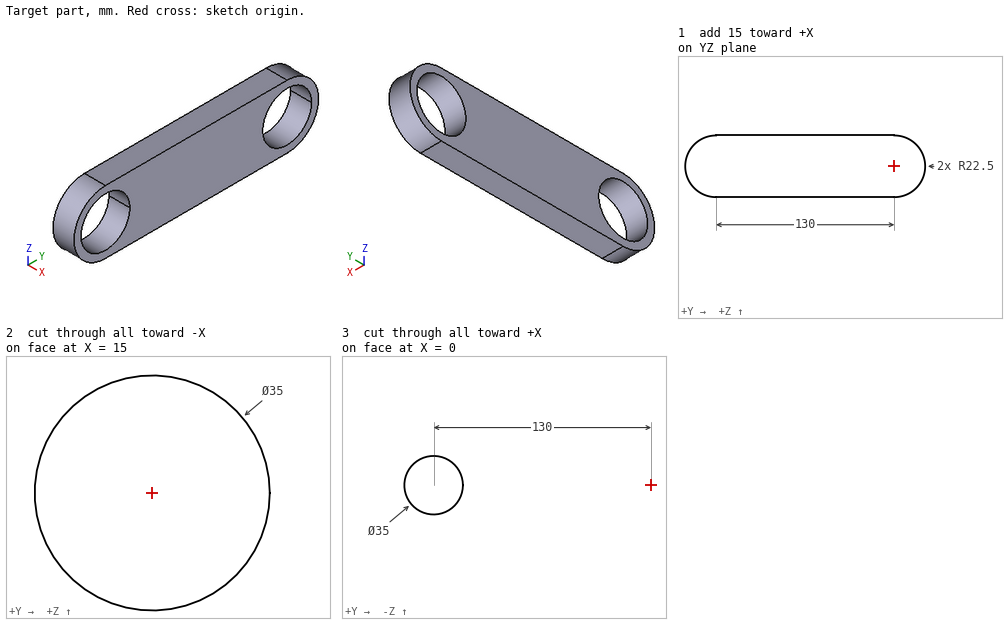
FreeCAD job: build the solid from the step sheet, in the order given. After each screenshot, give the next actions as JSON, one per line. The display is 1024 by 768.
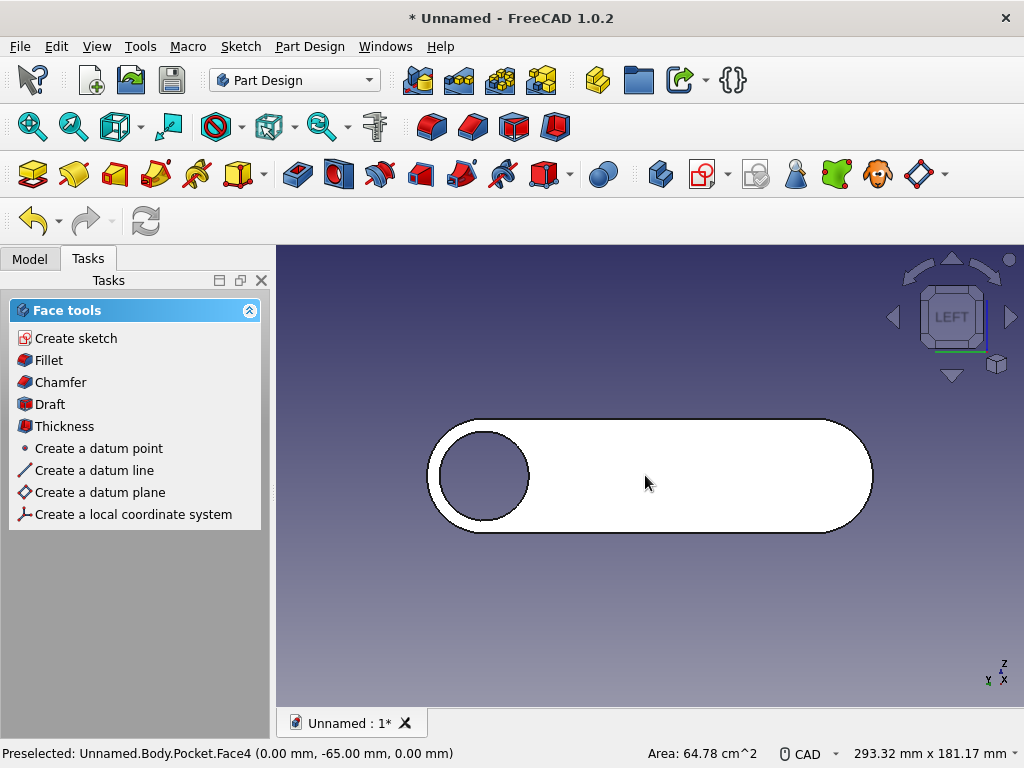
{"action": "left_click", "coordinate": [702, 174]}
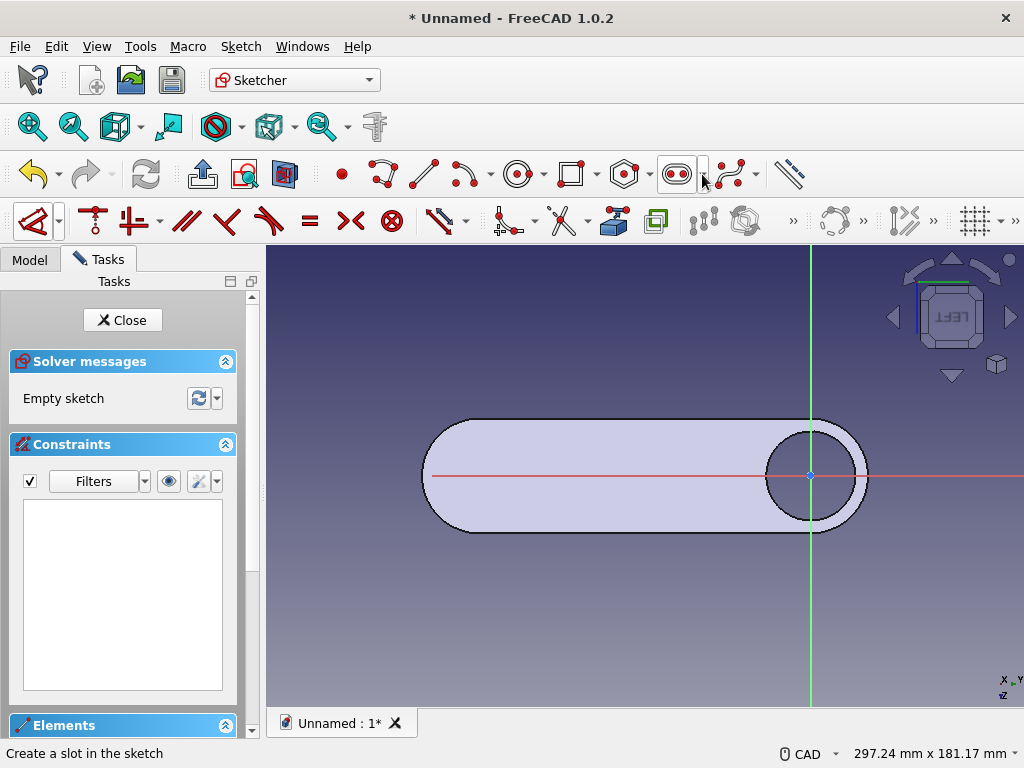
{"action": "scroll", "coordinate": [437, 476], "scroll_direction": "up", "scroll_amount": 6}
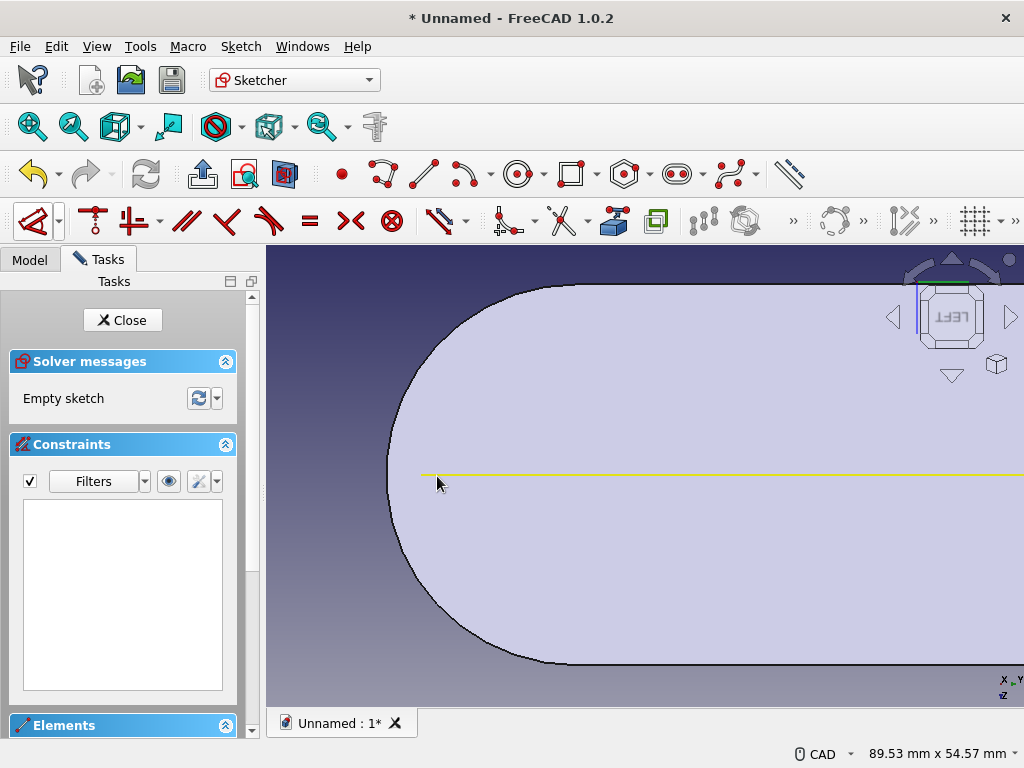
{"action": "left_click", "coordinate": [518, 174]}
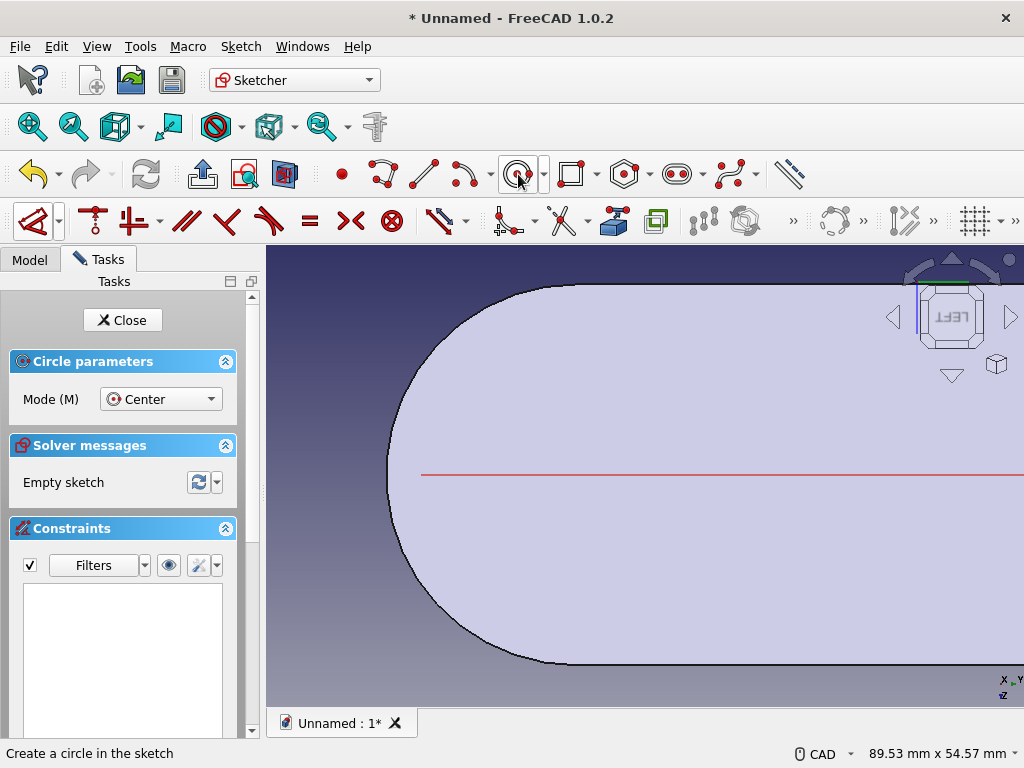
{"action": "left_click", "coordinate": [577, 475]}
{"action": "left_click", "coordinate": [681, 370]}
{"action": "key", "text": "Escape"}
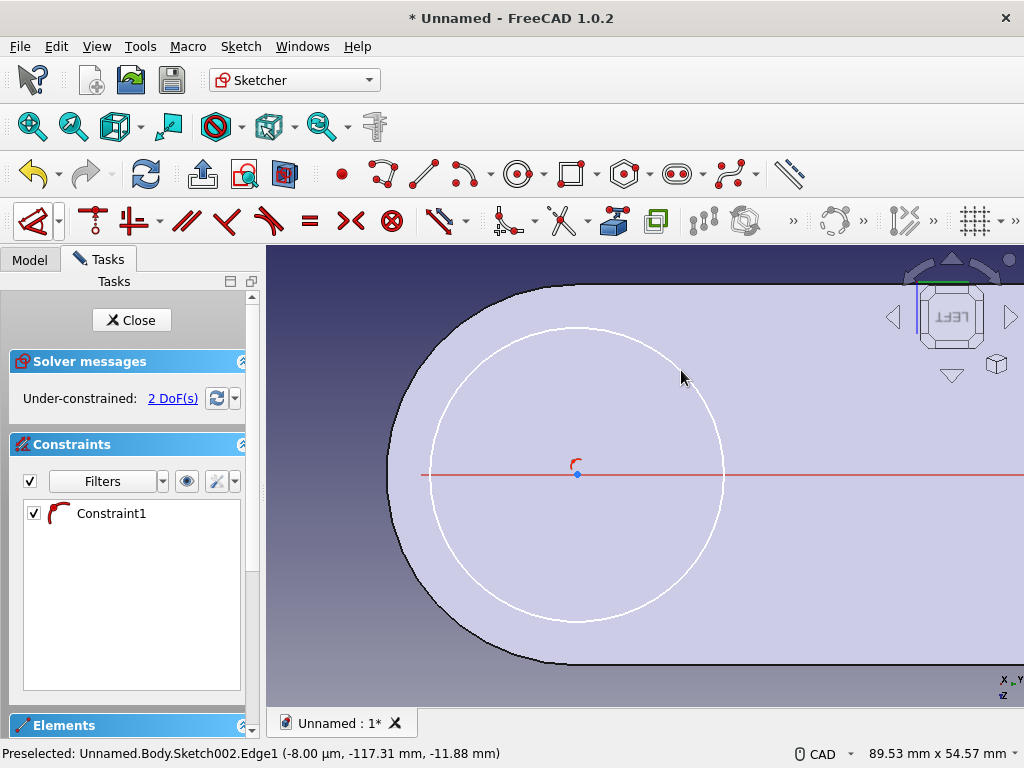
{"action": "left_click", "coordinate": [681, 371]}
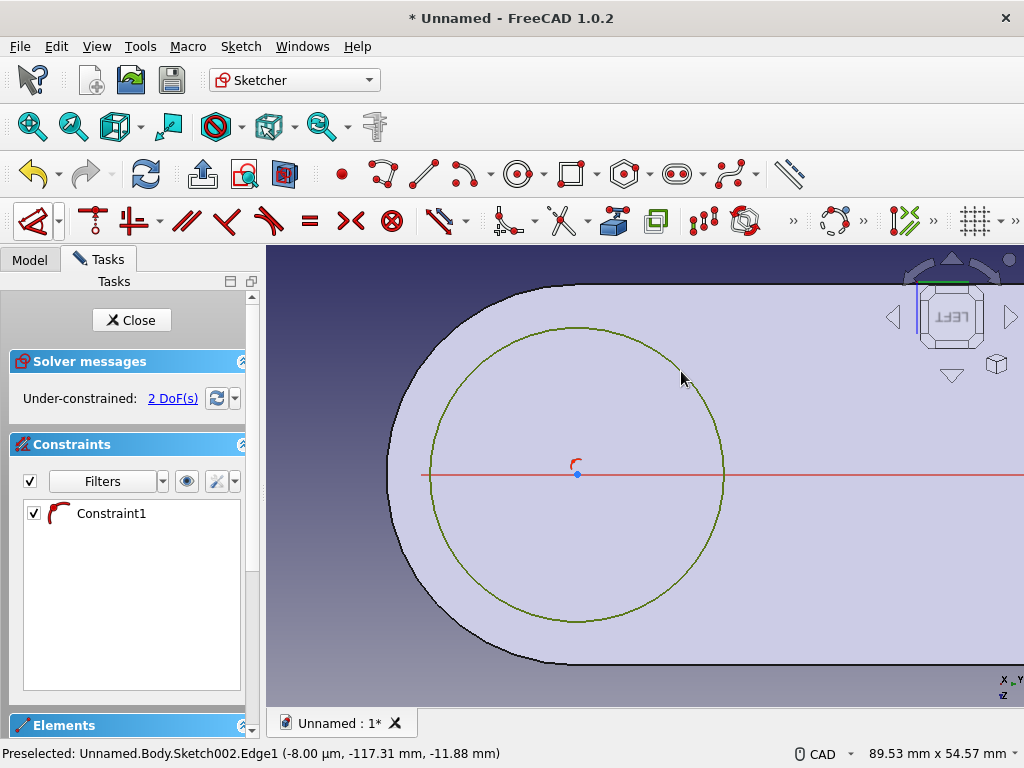
{"action": "key", "text": "k o"}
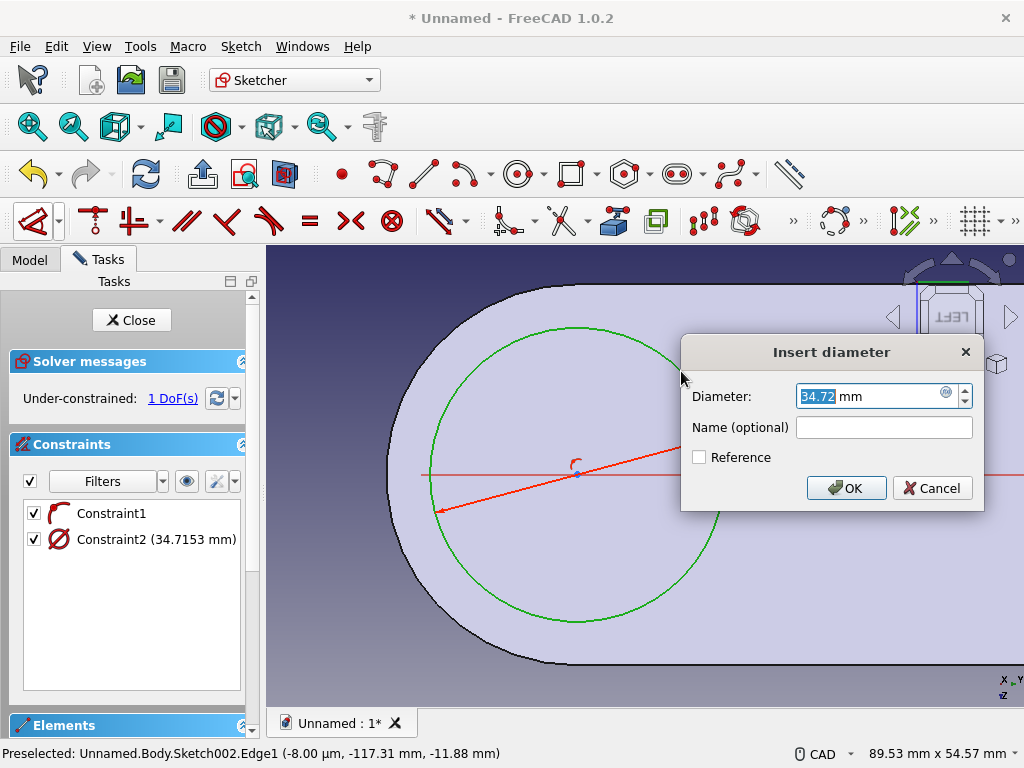
{"action": "type", "text": "35"}
{"action": "key", "text": "Return"}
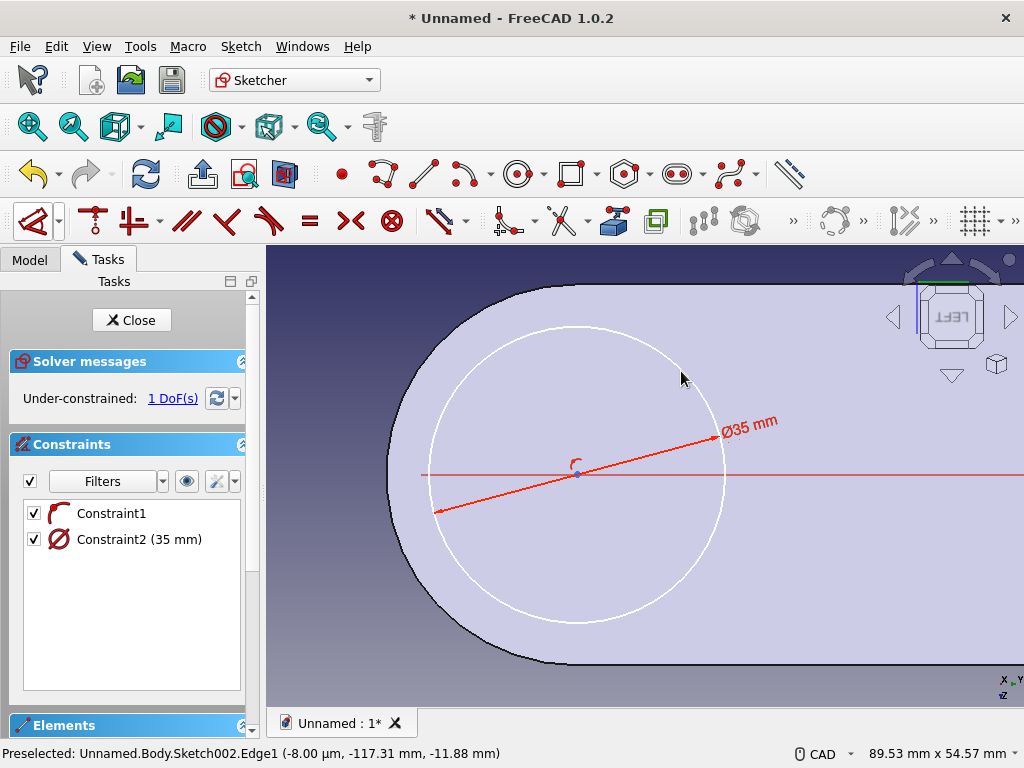
{"action": "left_click", "coordinate": [577, 475]}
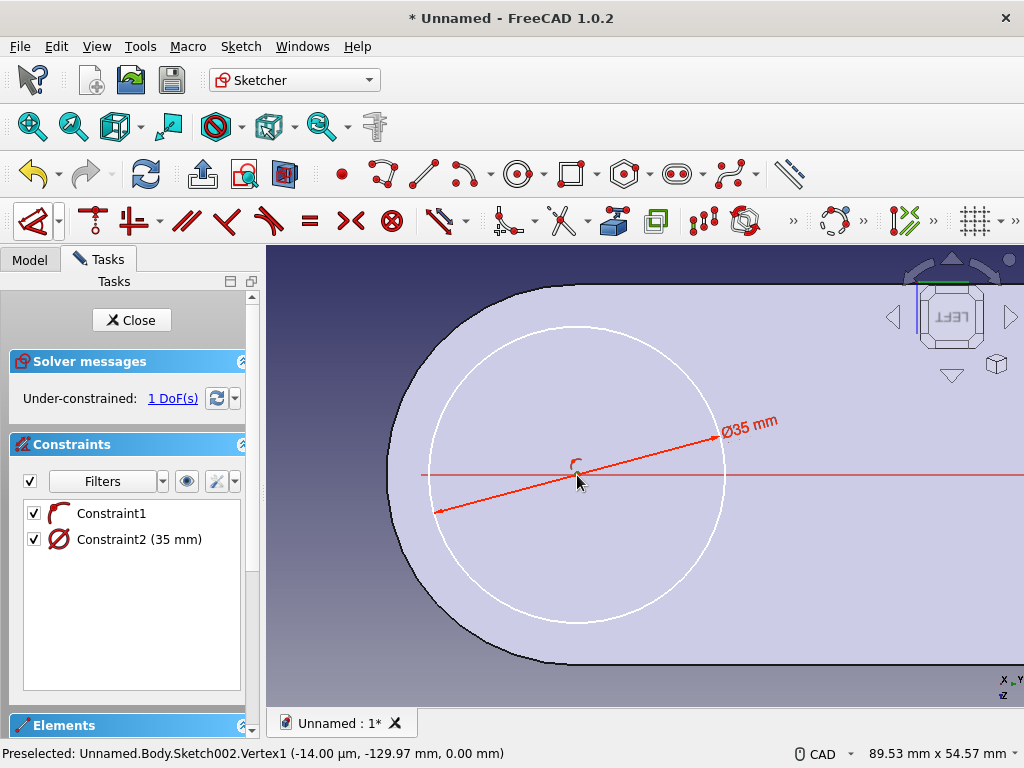
{"action": "left_click", "coordinate": [58, 222]}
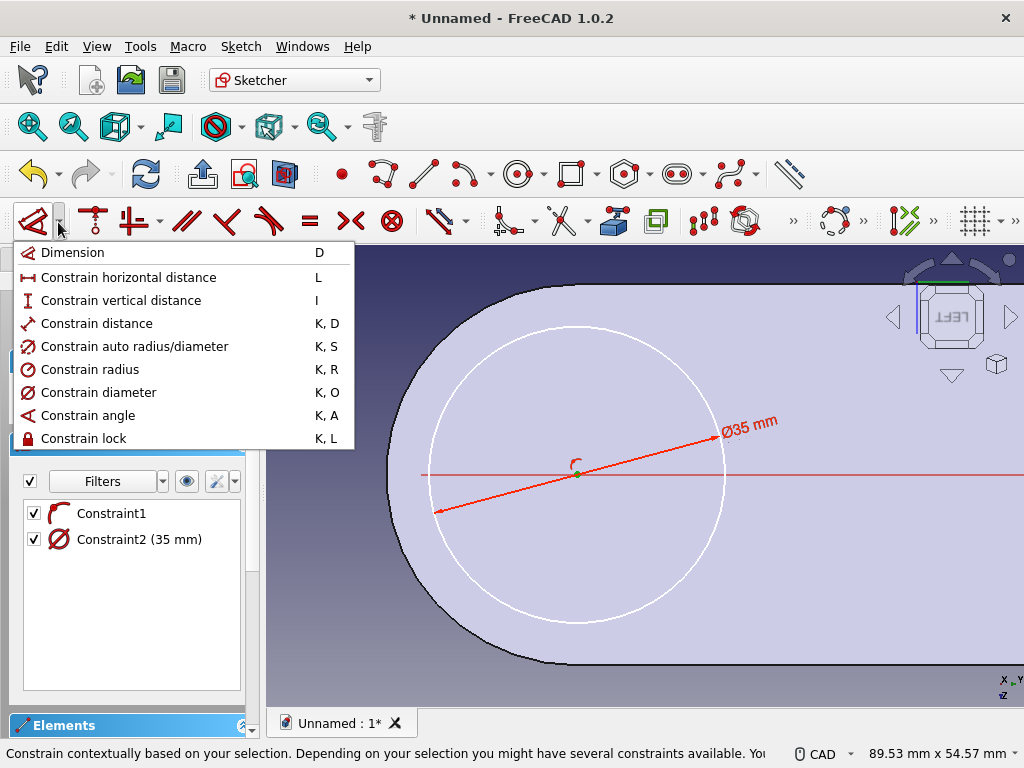
{"action": "left_click", "coordinate": [184, 278]}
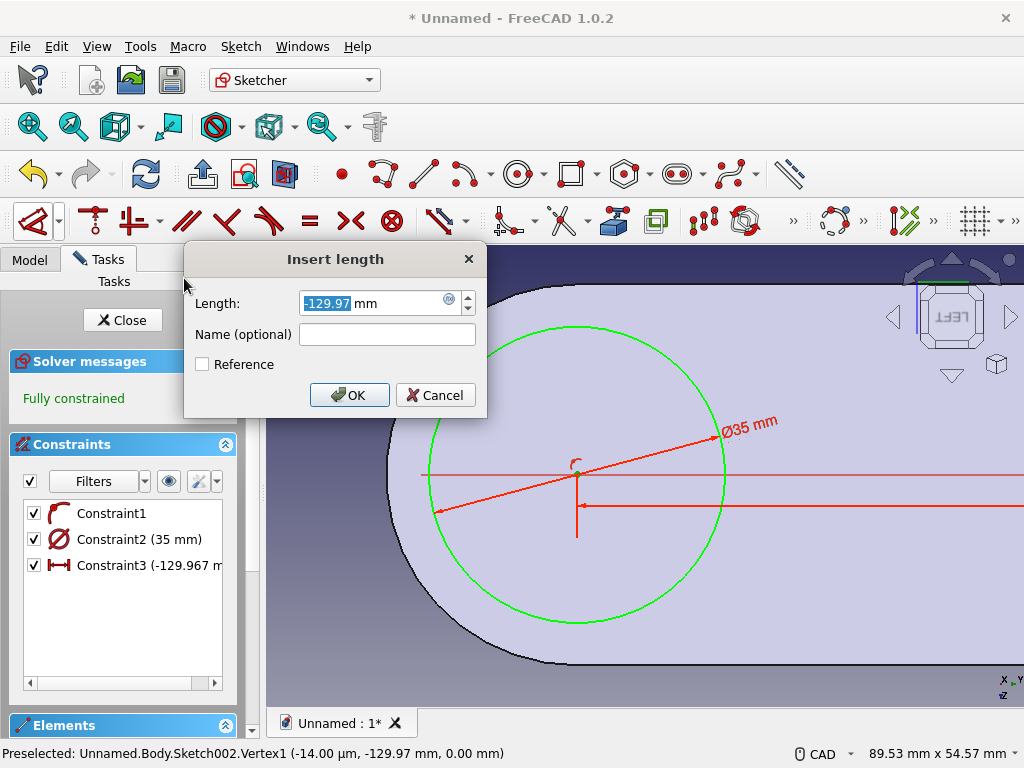
{"action": "type", "text": "-130"}
{"action": "key", "text": "Return"}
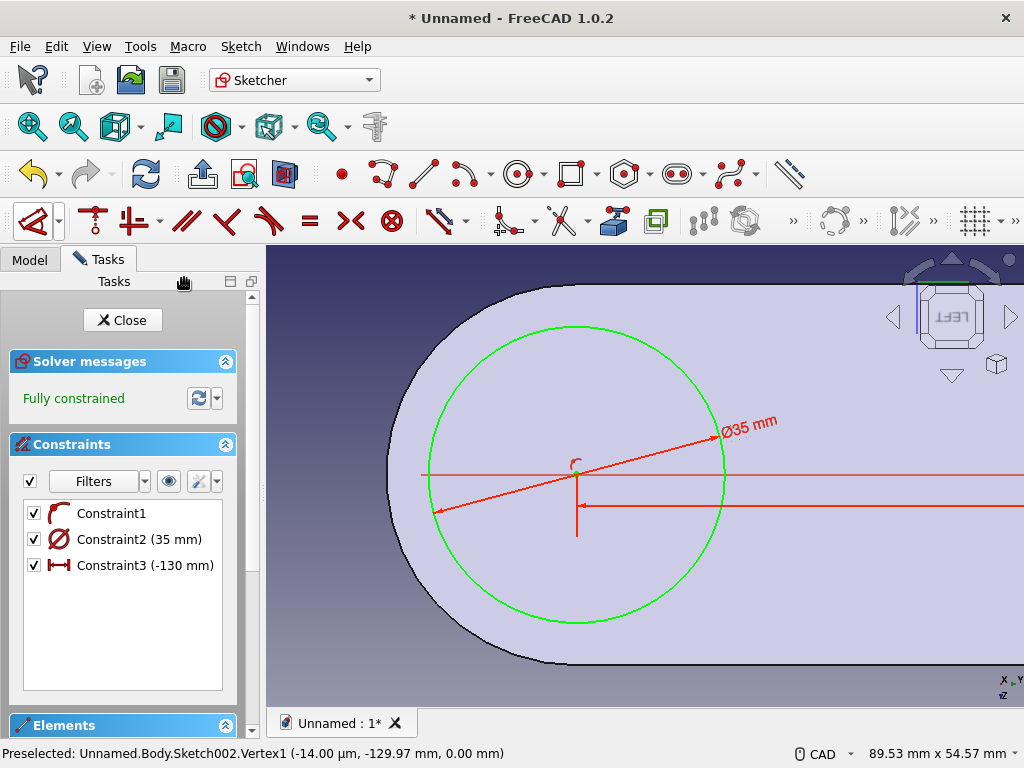
{"action": "left_click", "coordinate": [123, 320]}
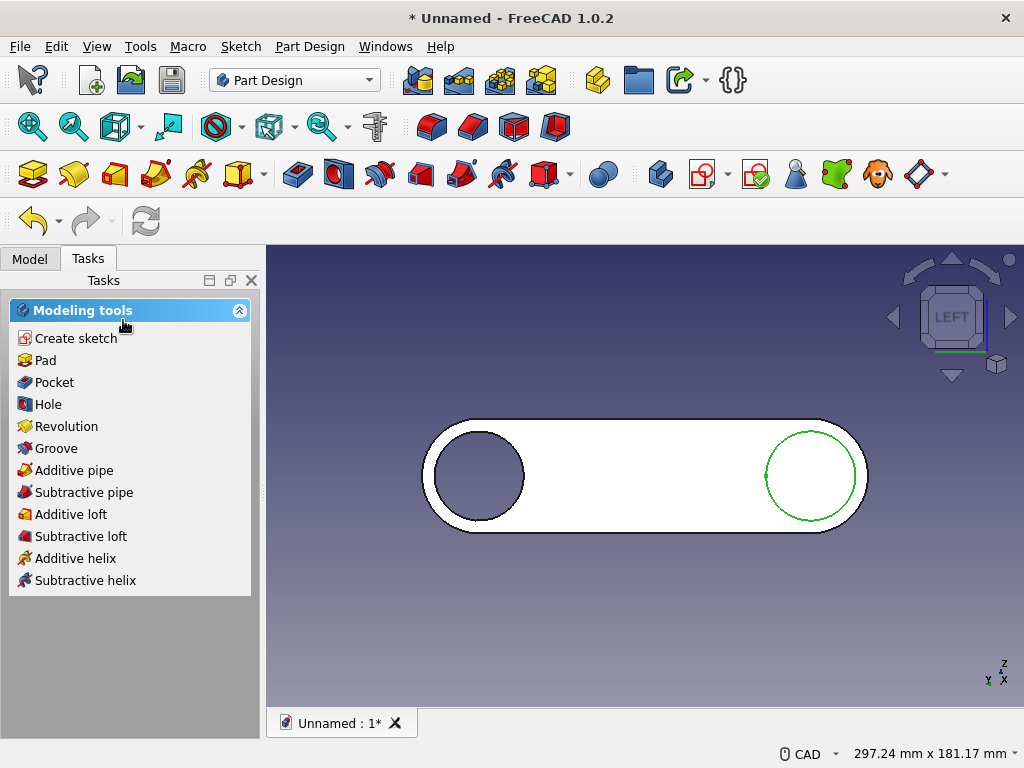
{"action": "left_click", "coordinate": [298, 174]}